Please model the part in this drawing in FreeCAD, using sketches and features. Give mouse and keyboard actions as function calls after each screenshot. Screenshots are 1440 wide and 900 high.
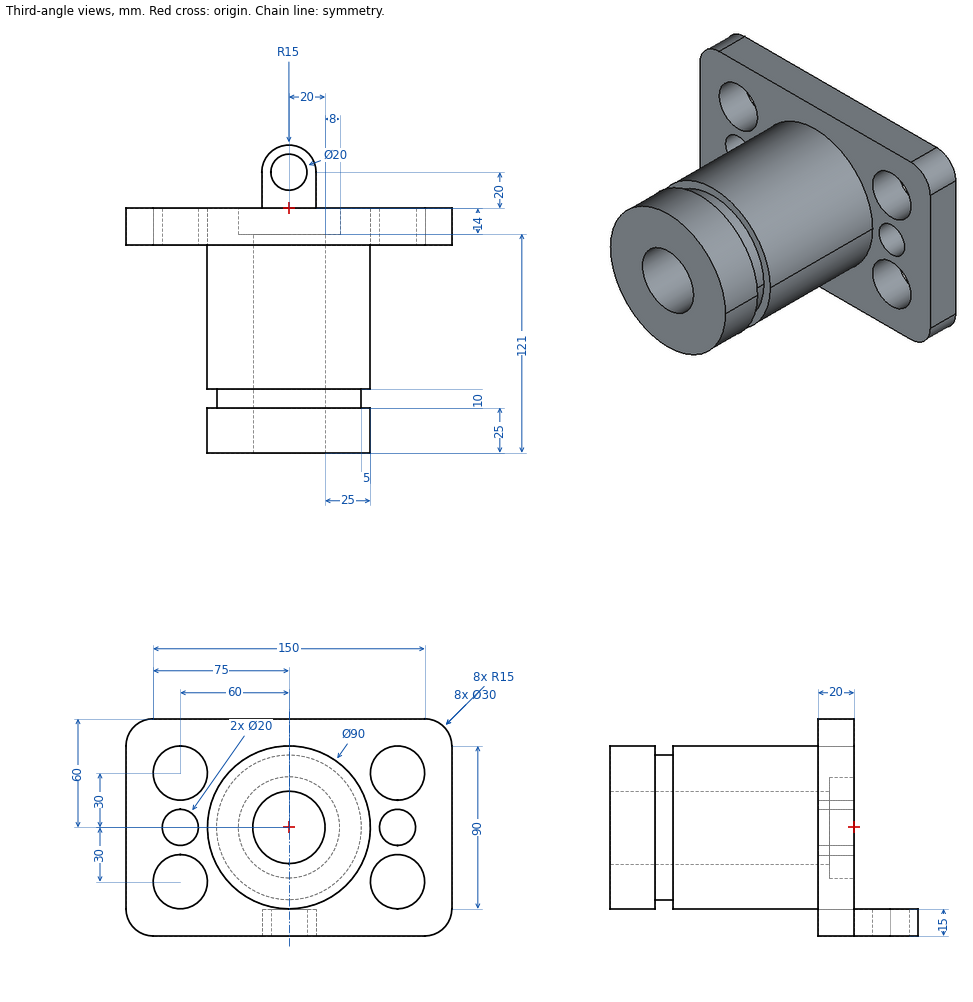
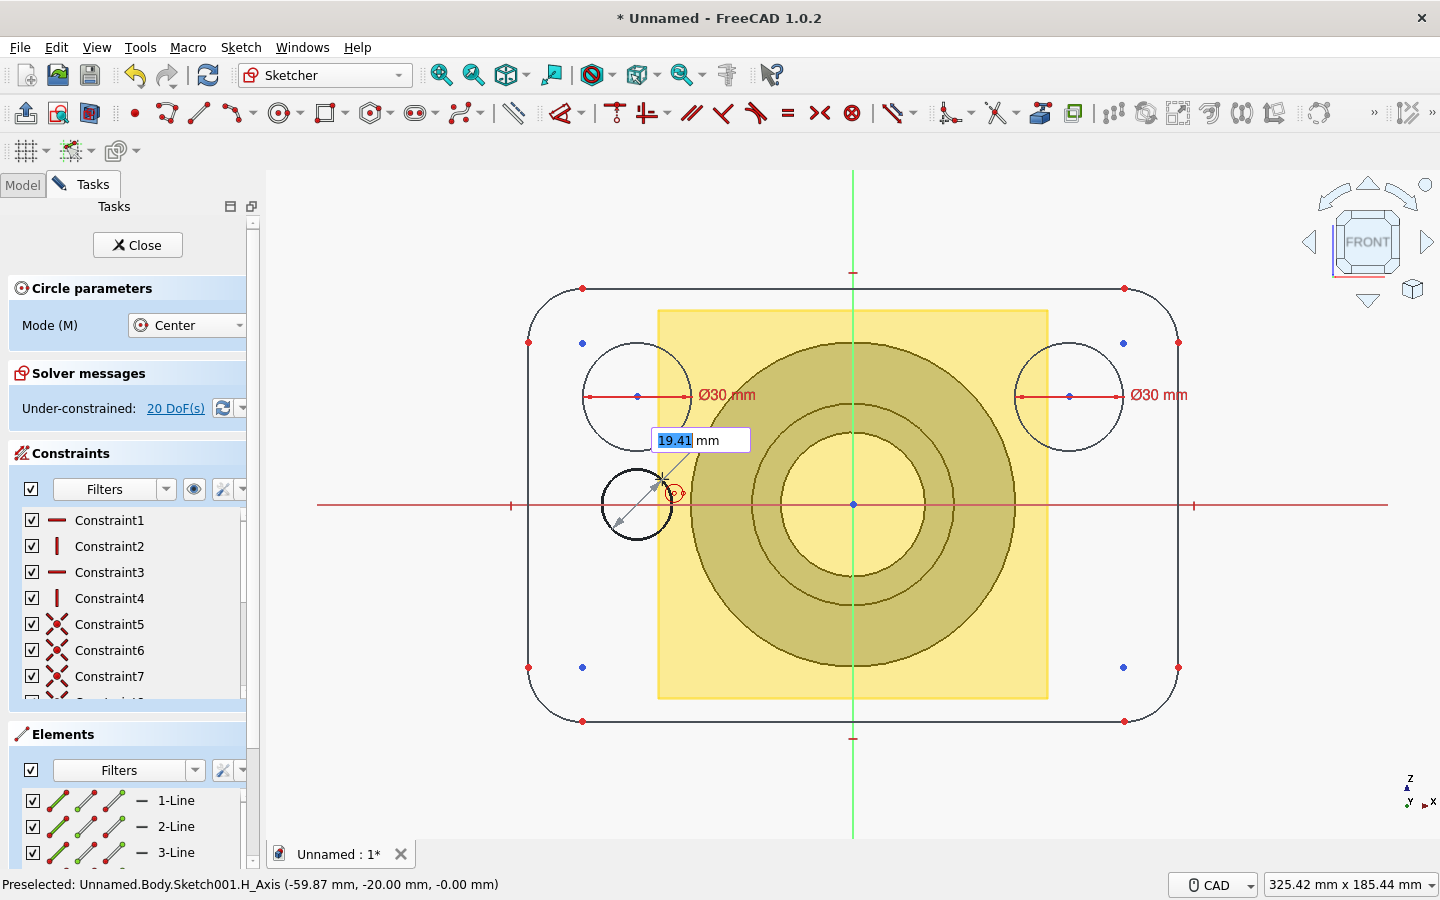
text(20)
key(Return)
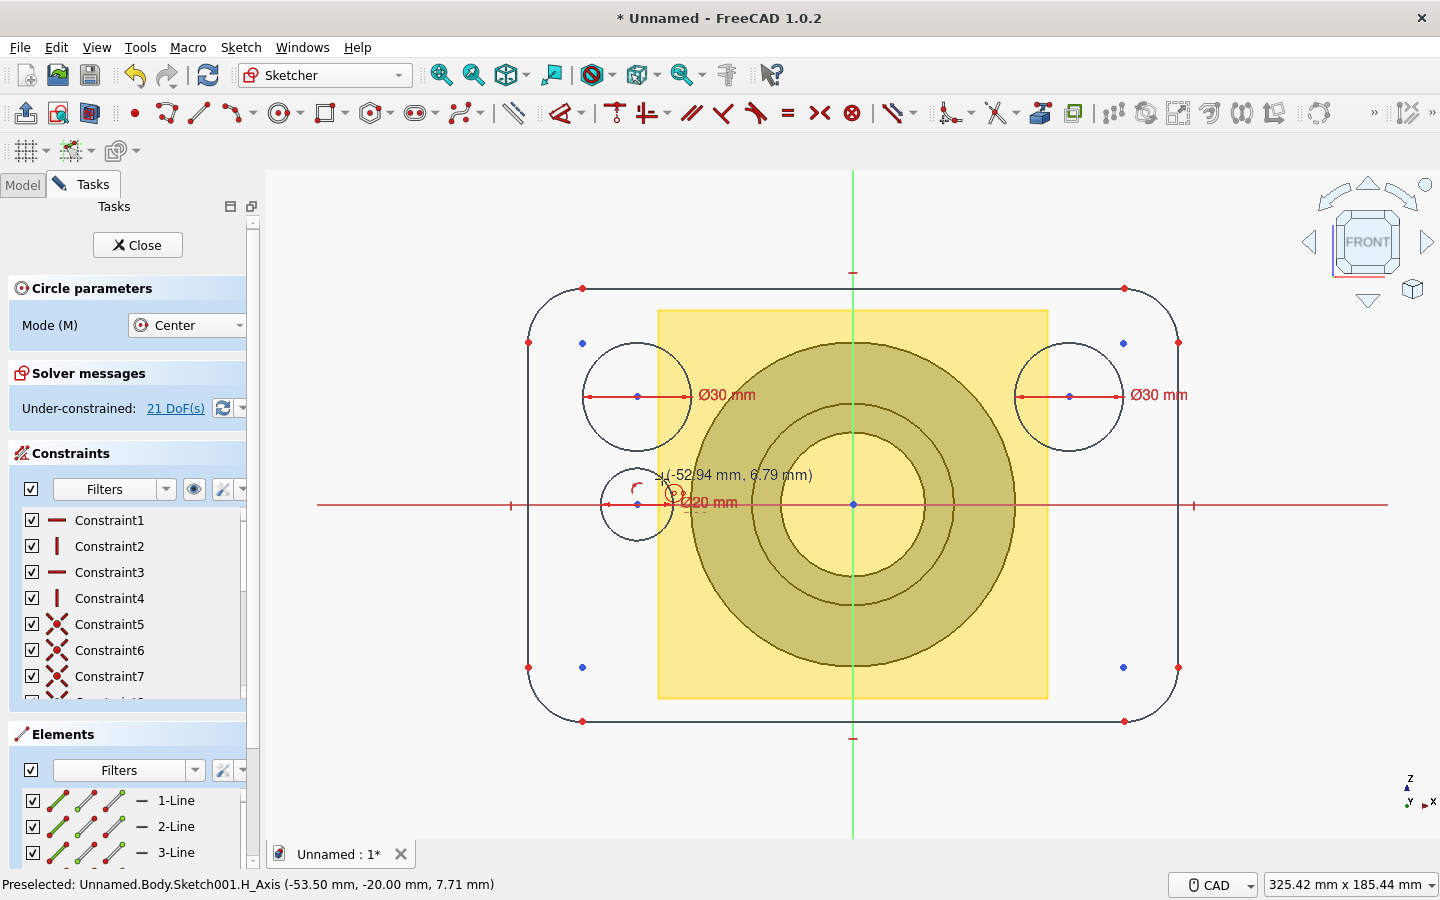
click(637, 613)
move(675, 574)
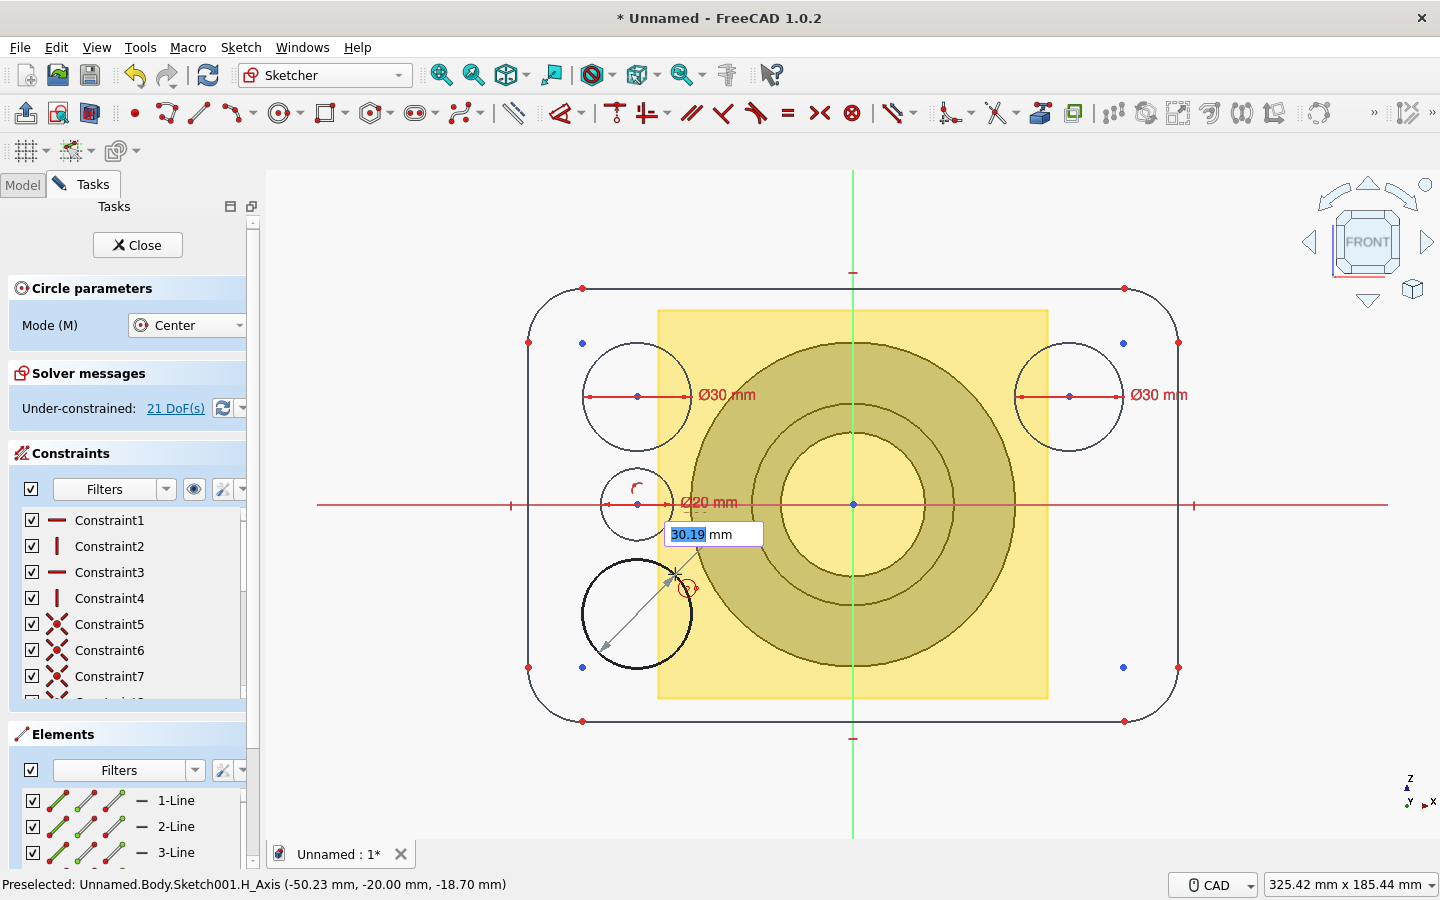
text(30)
key(Return)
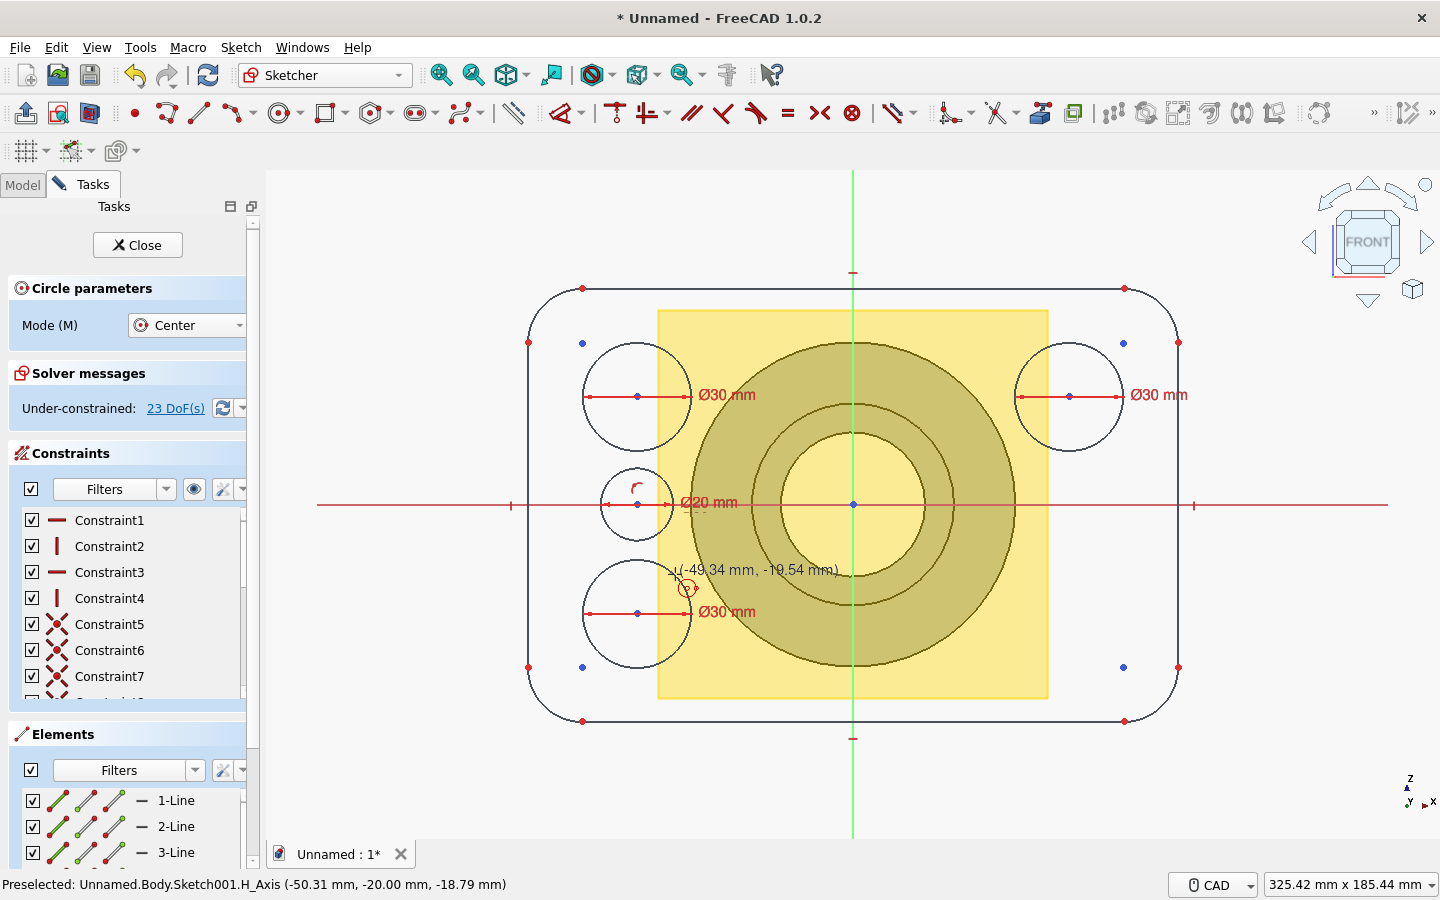
click(853, 504)
move(968, 390)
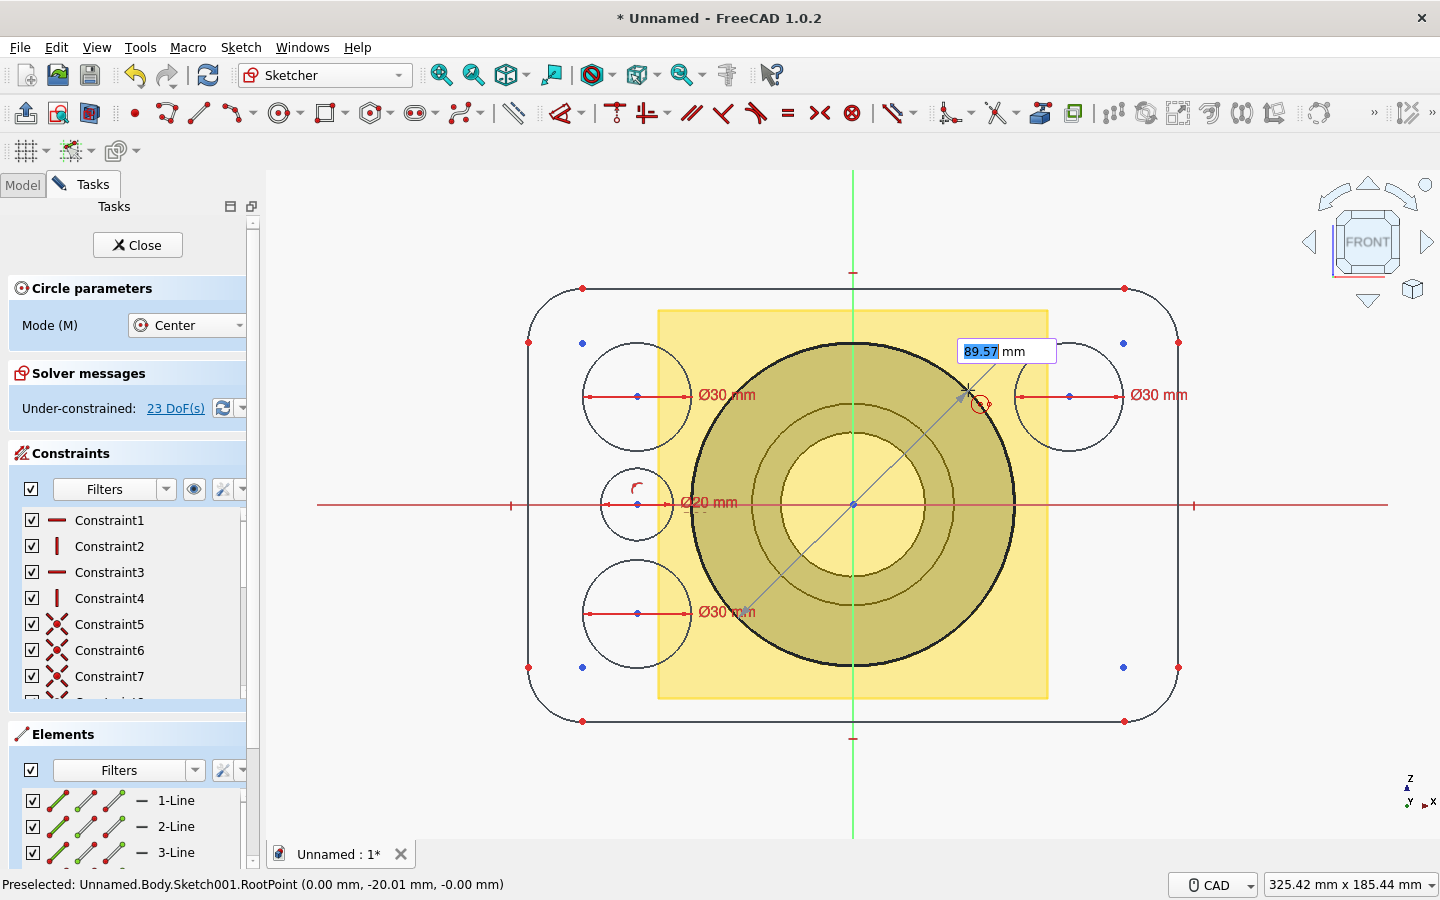
text(90)
key(Return)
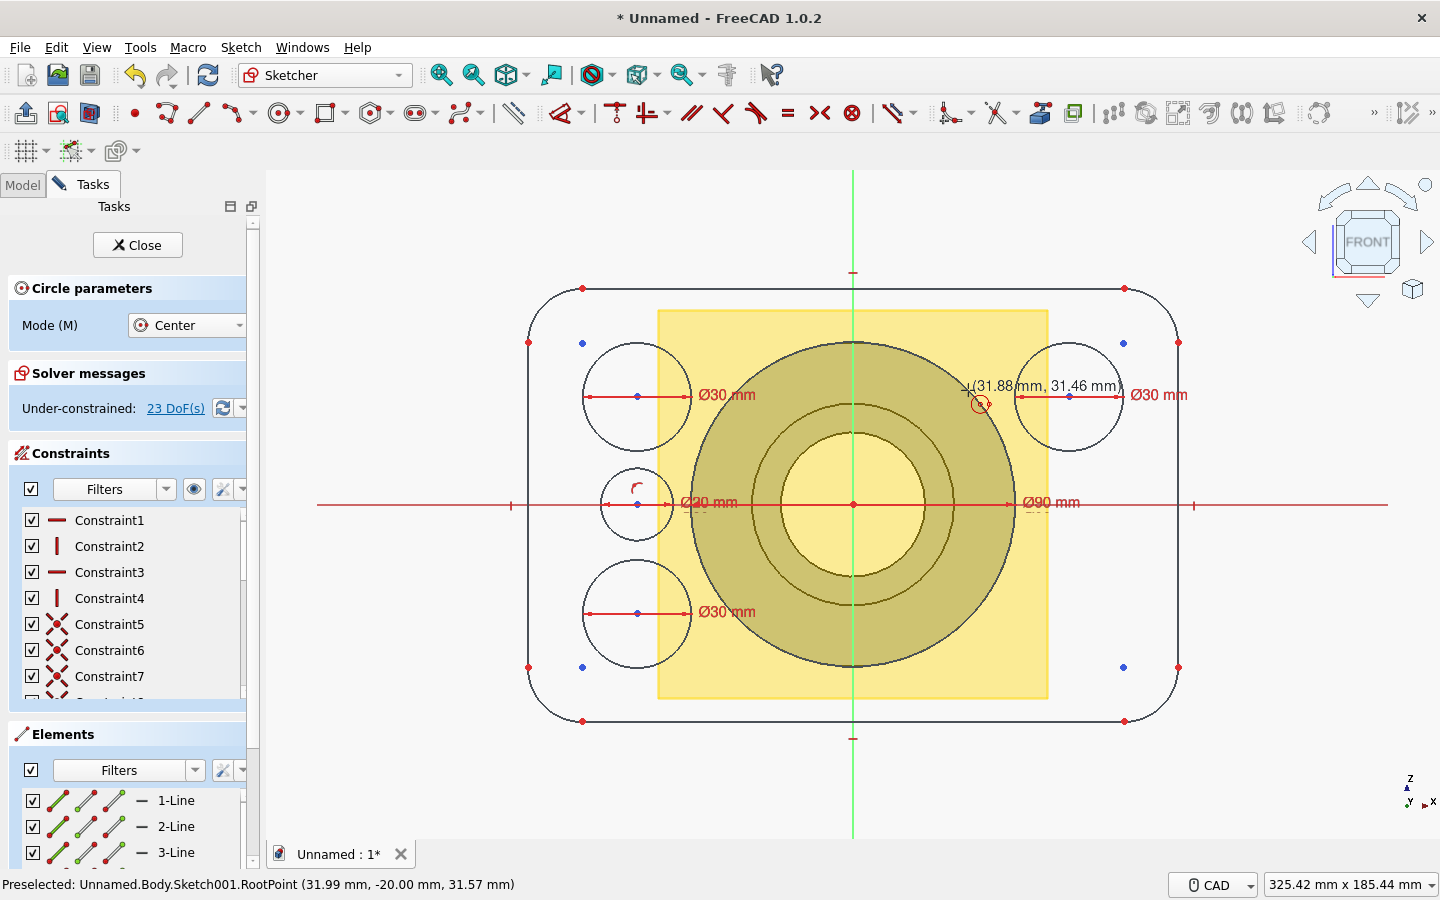
click(1069, 504)
move(1095, 479)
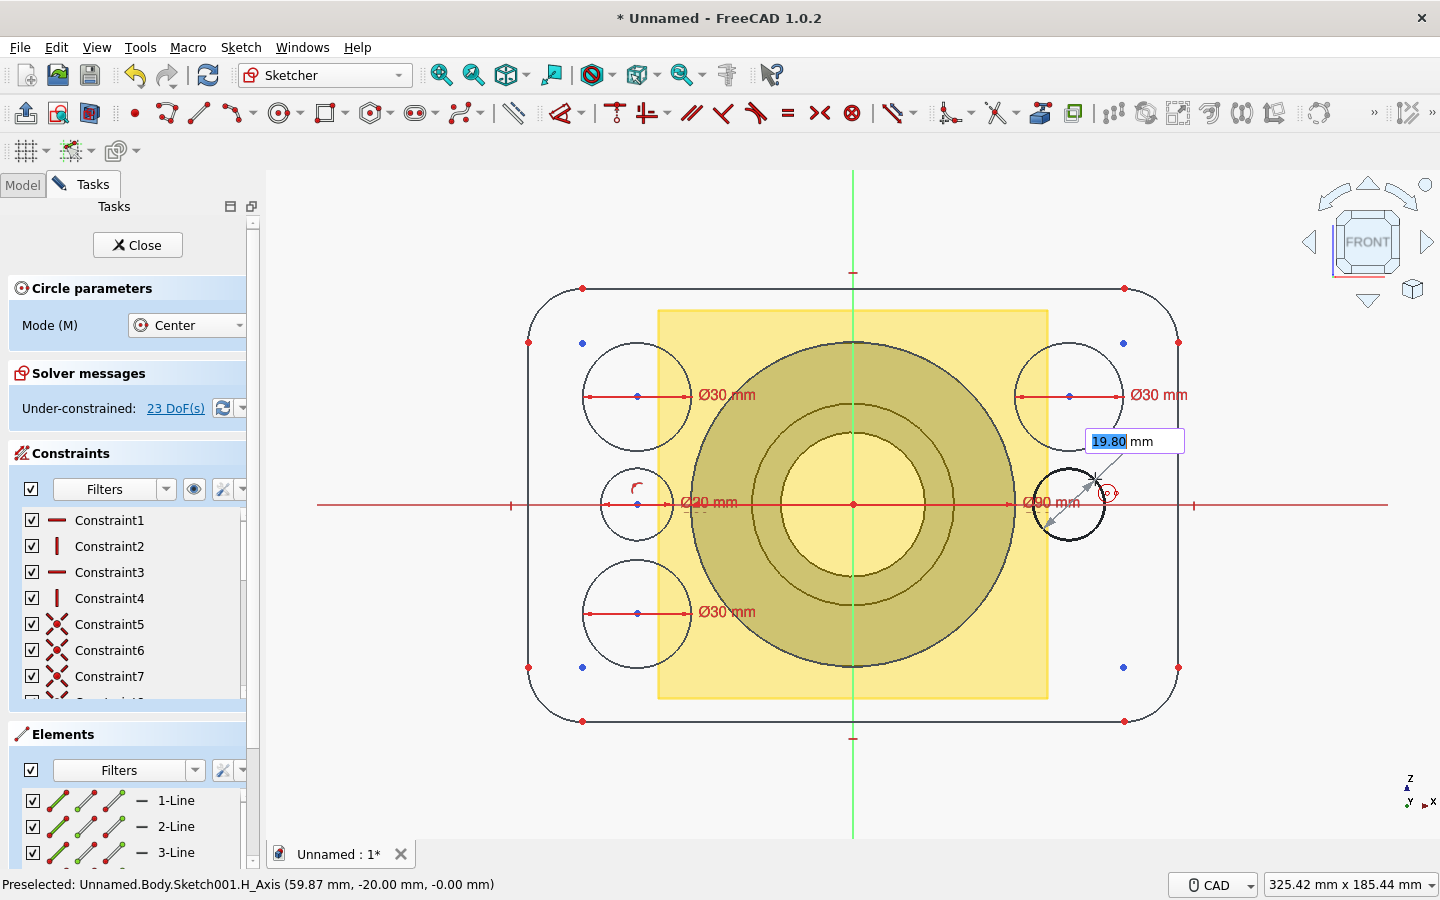
text(20)
key(Return)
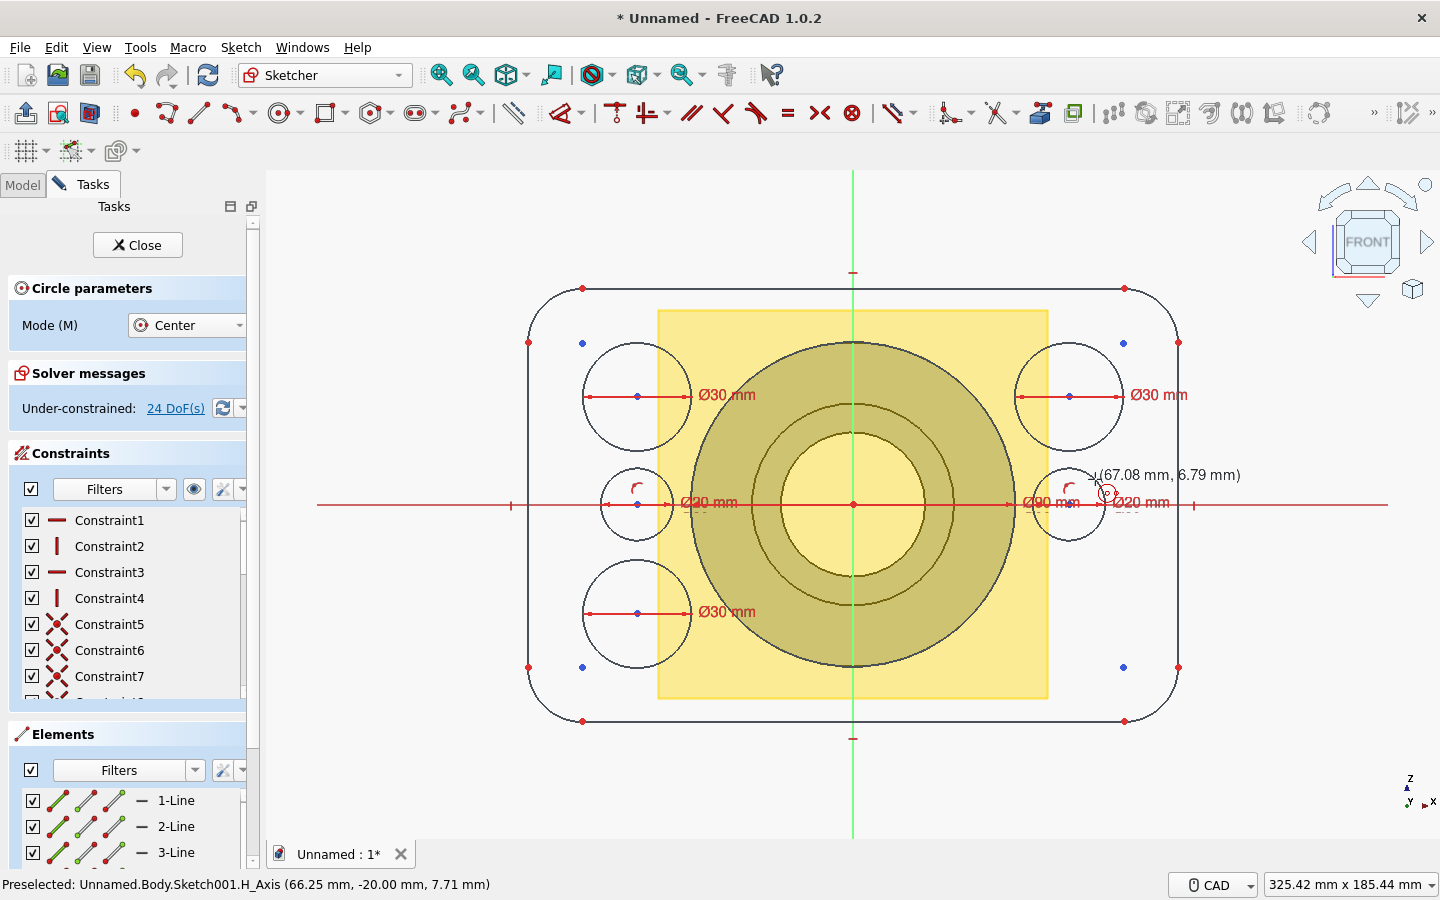
click(1069, 613)
move(1108, 574)